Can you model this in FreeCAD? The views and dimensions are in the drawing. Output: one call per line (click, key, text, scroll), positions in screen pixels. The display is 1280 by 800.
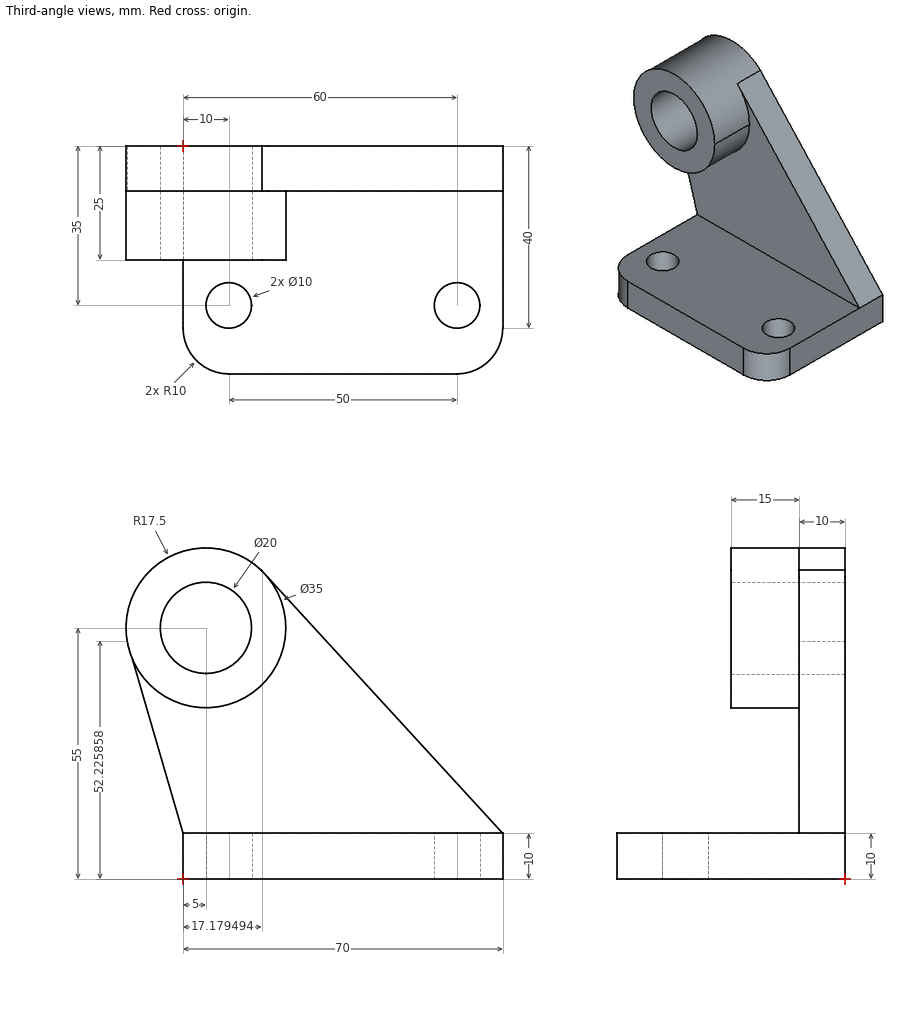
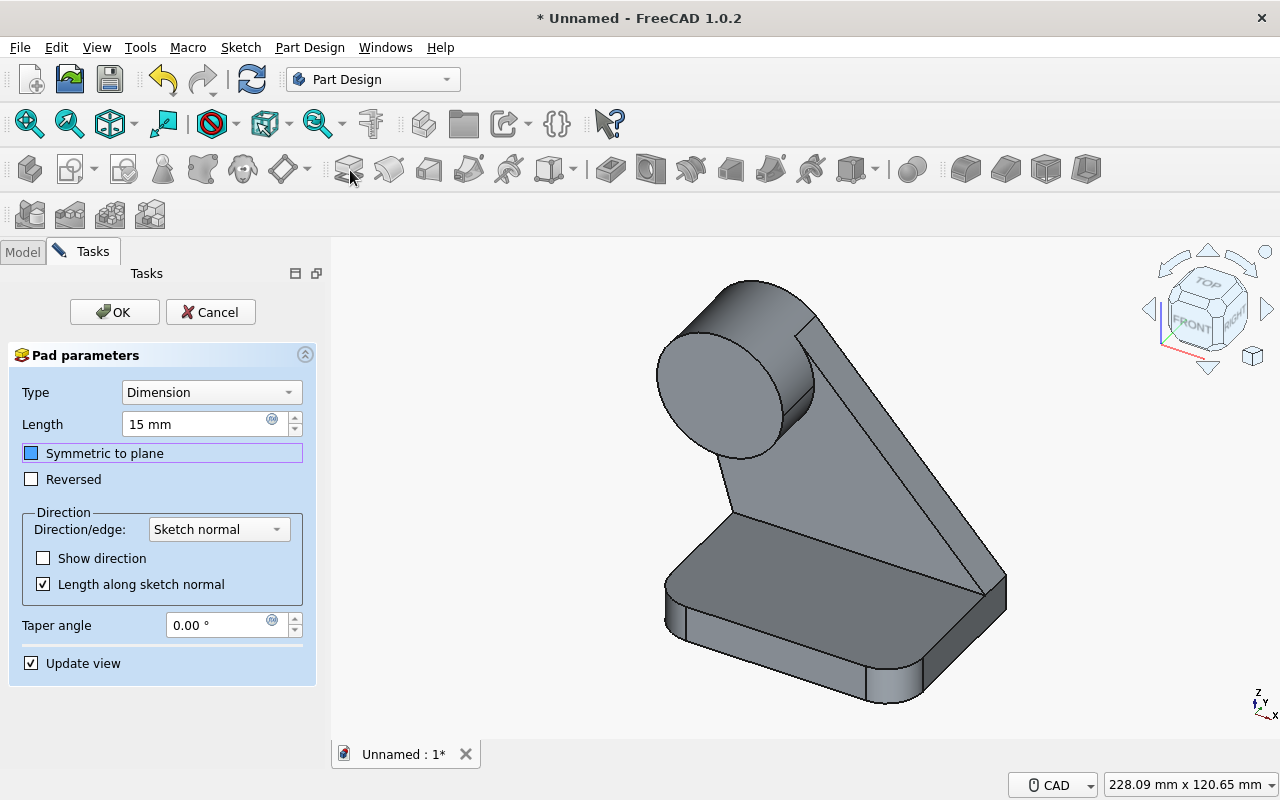
click(115, 312)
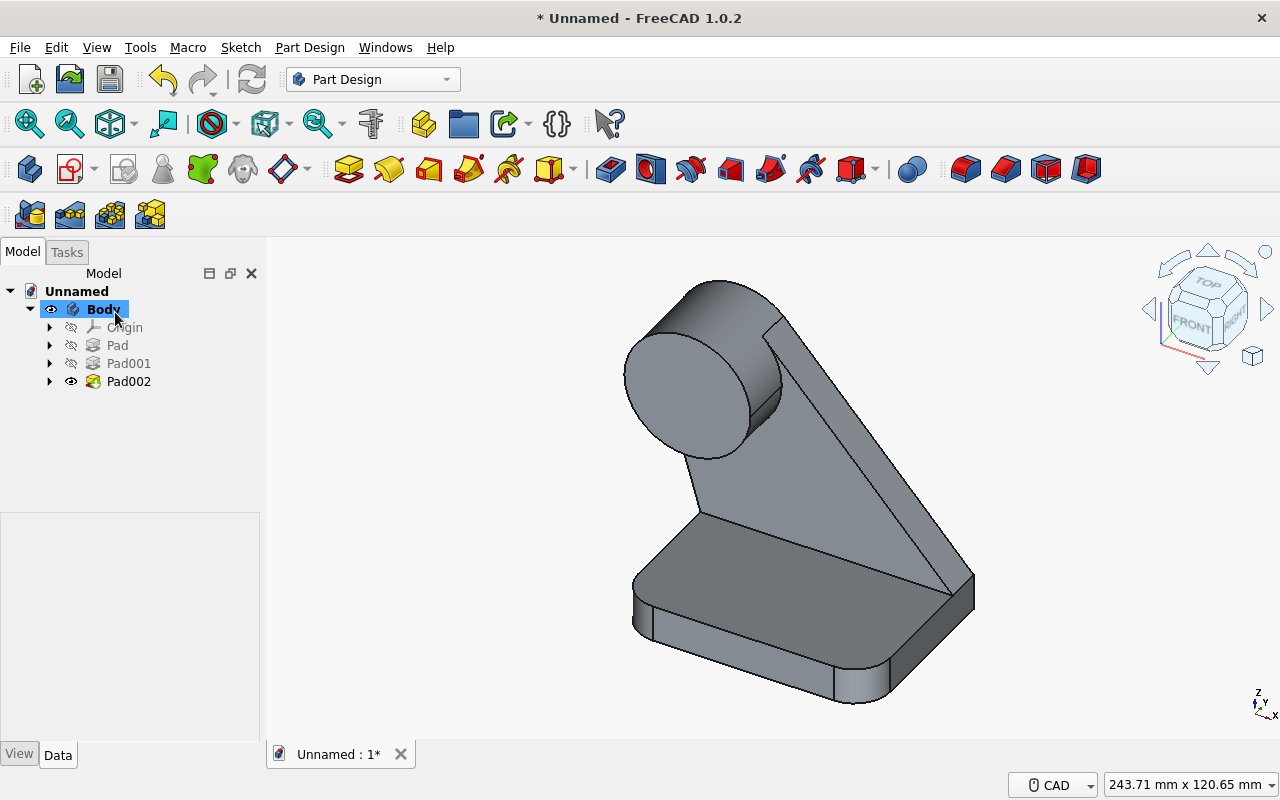
click(687, 395)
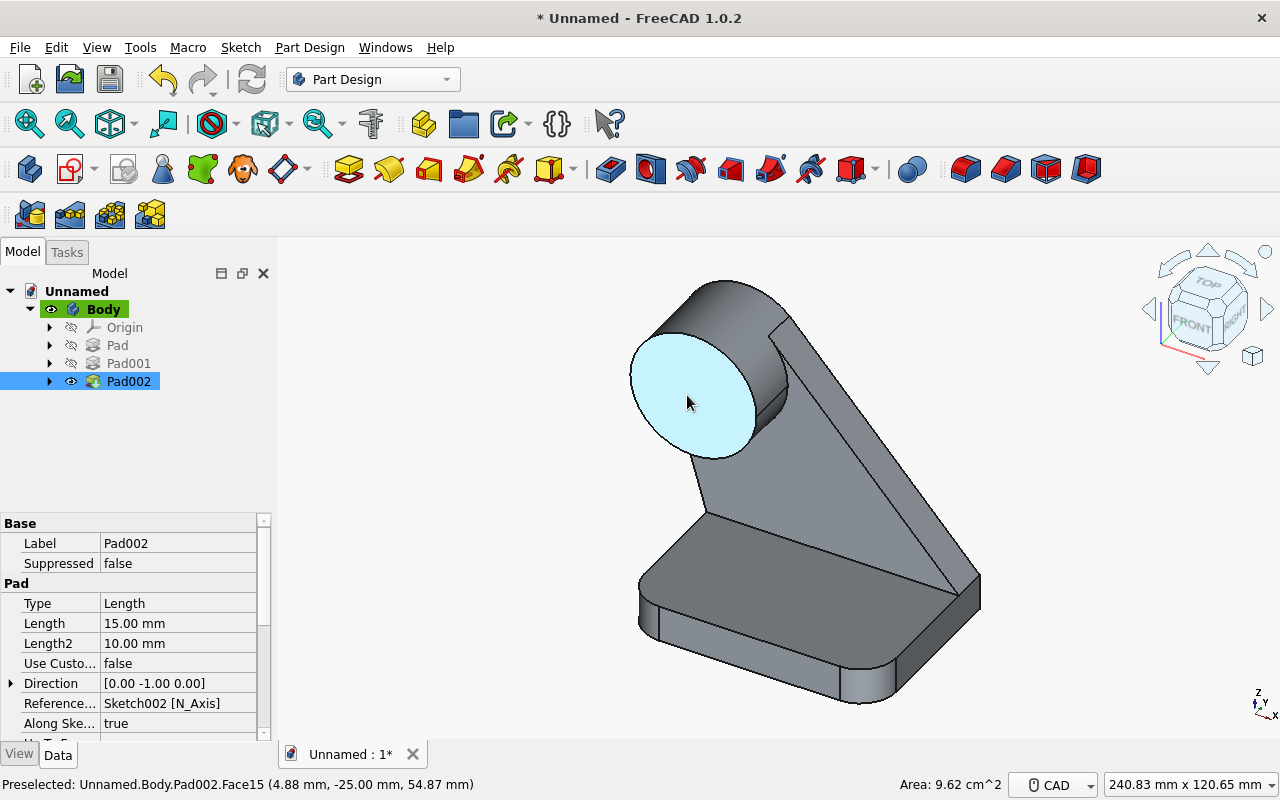
click(70, 170)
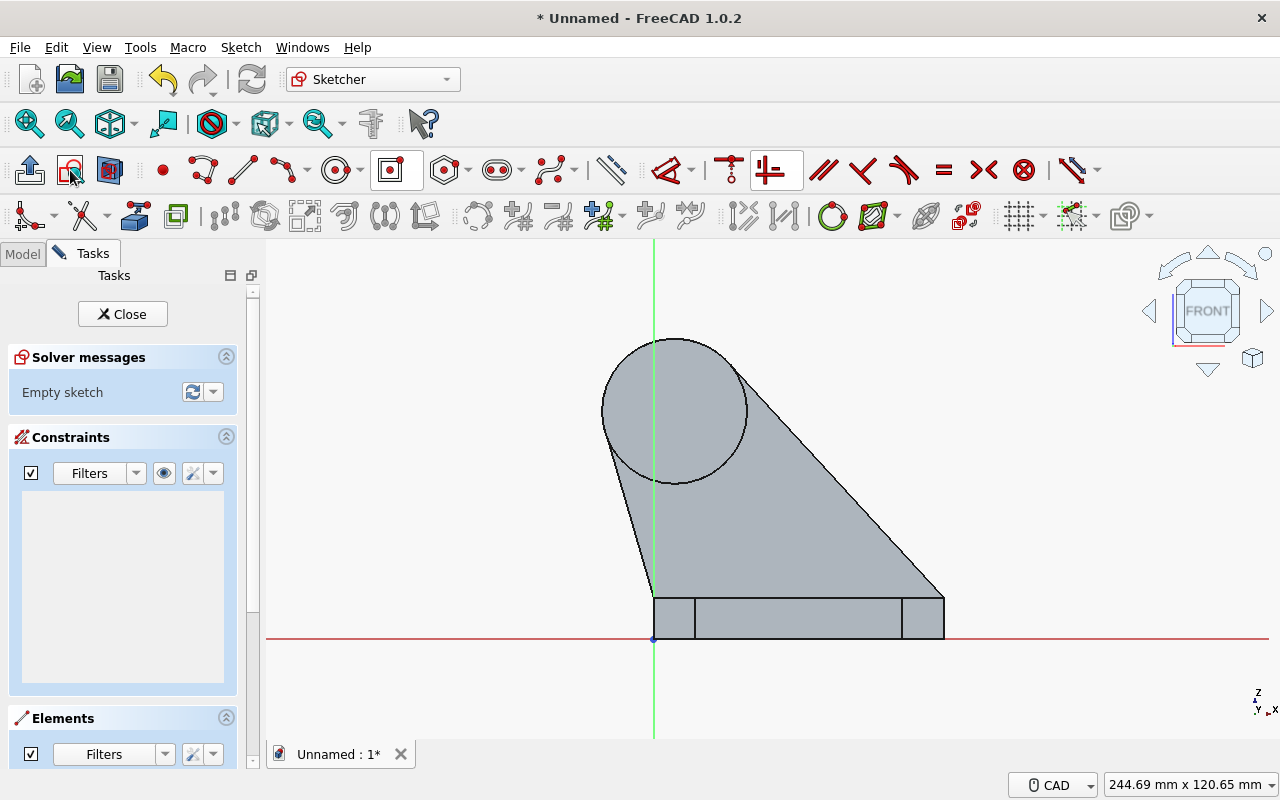
click(110, 170)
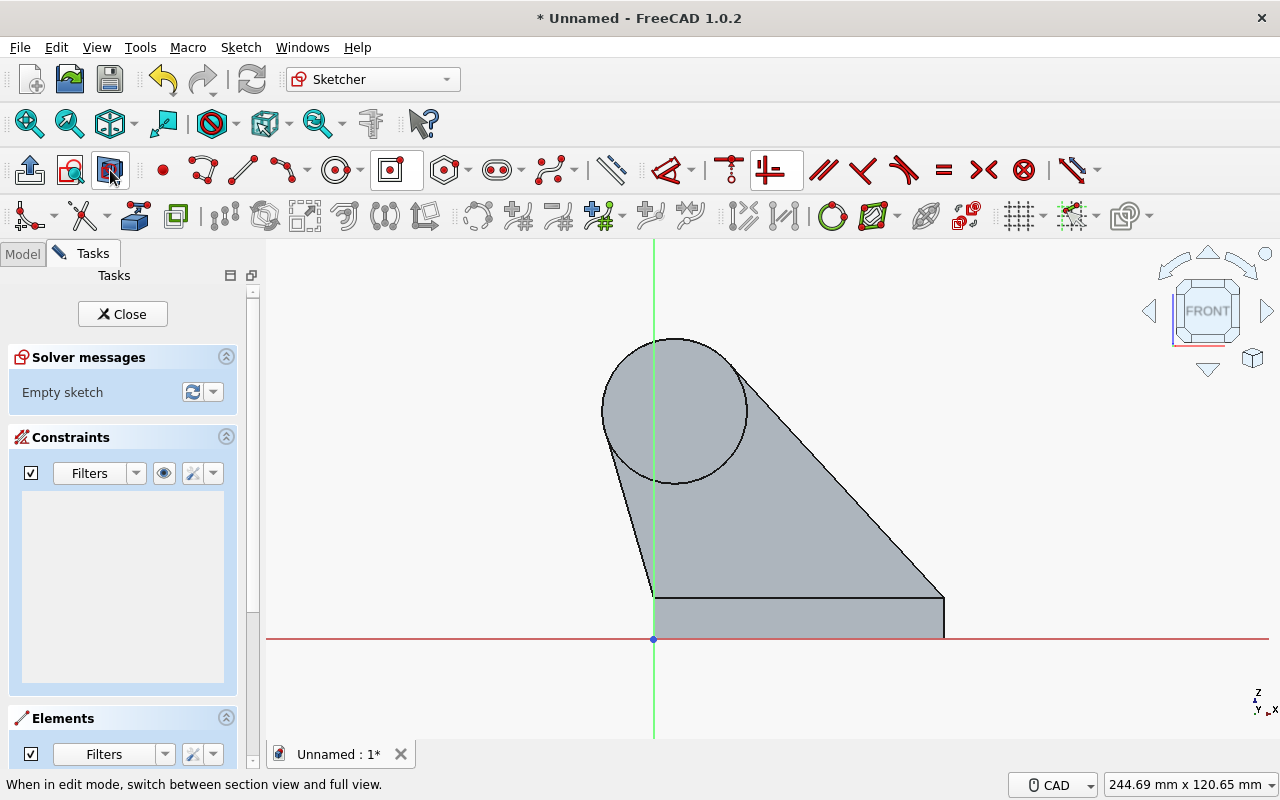
scroll(665, 386, up, 7)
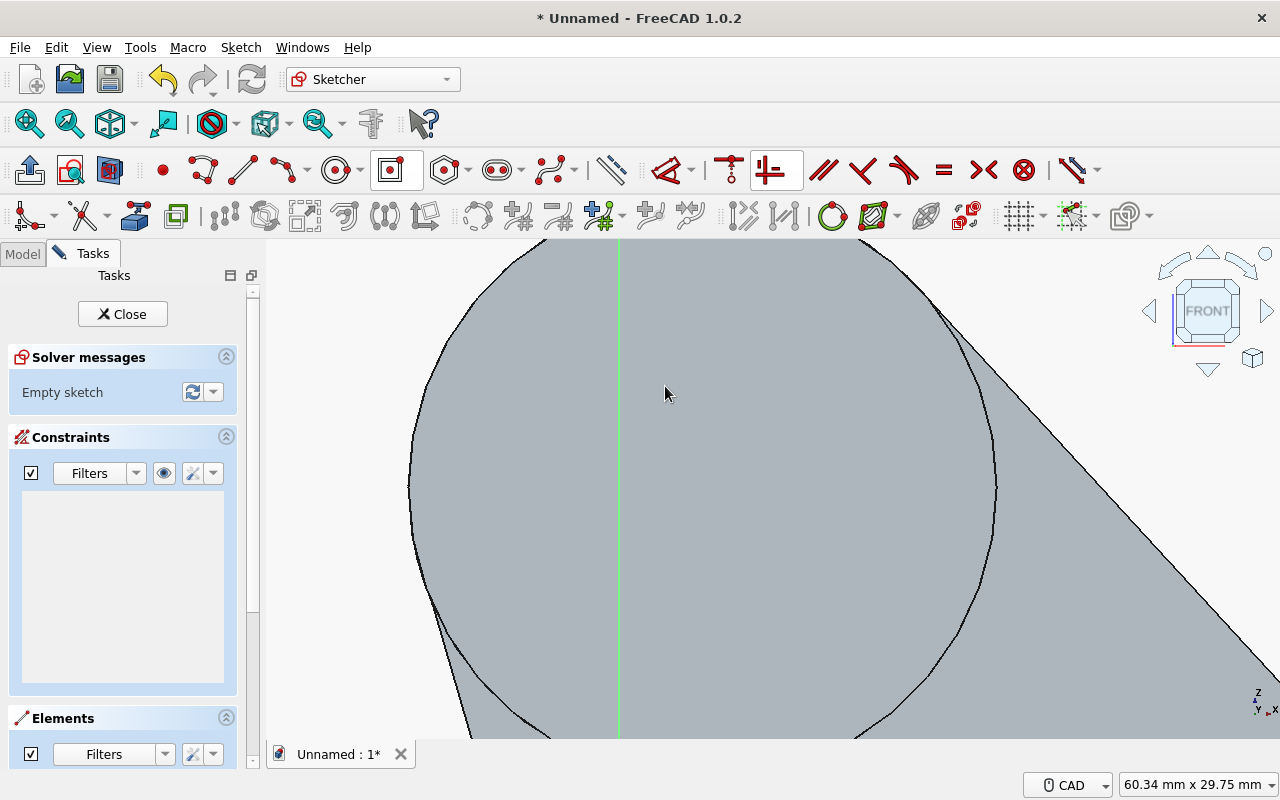
click(336, 170)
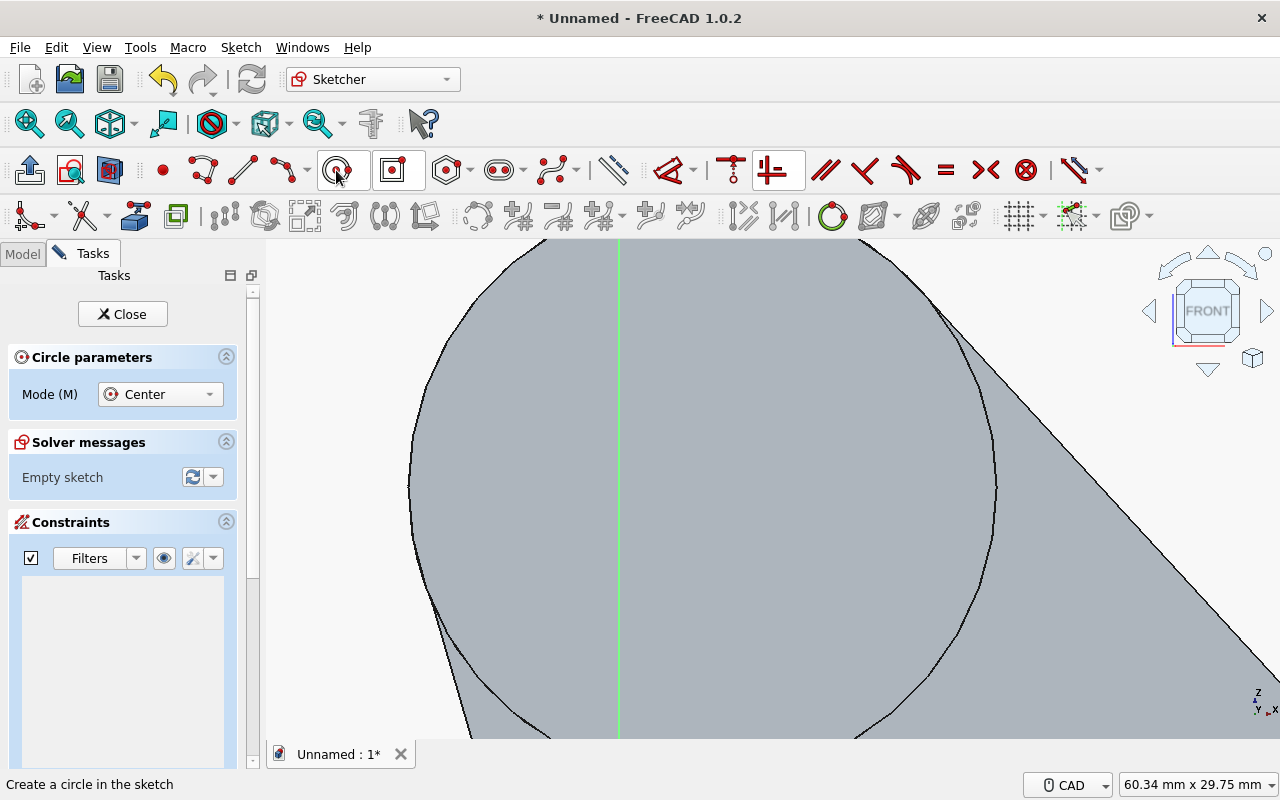
click(703, 487)
click(821, 369)
key(Escape)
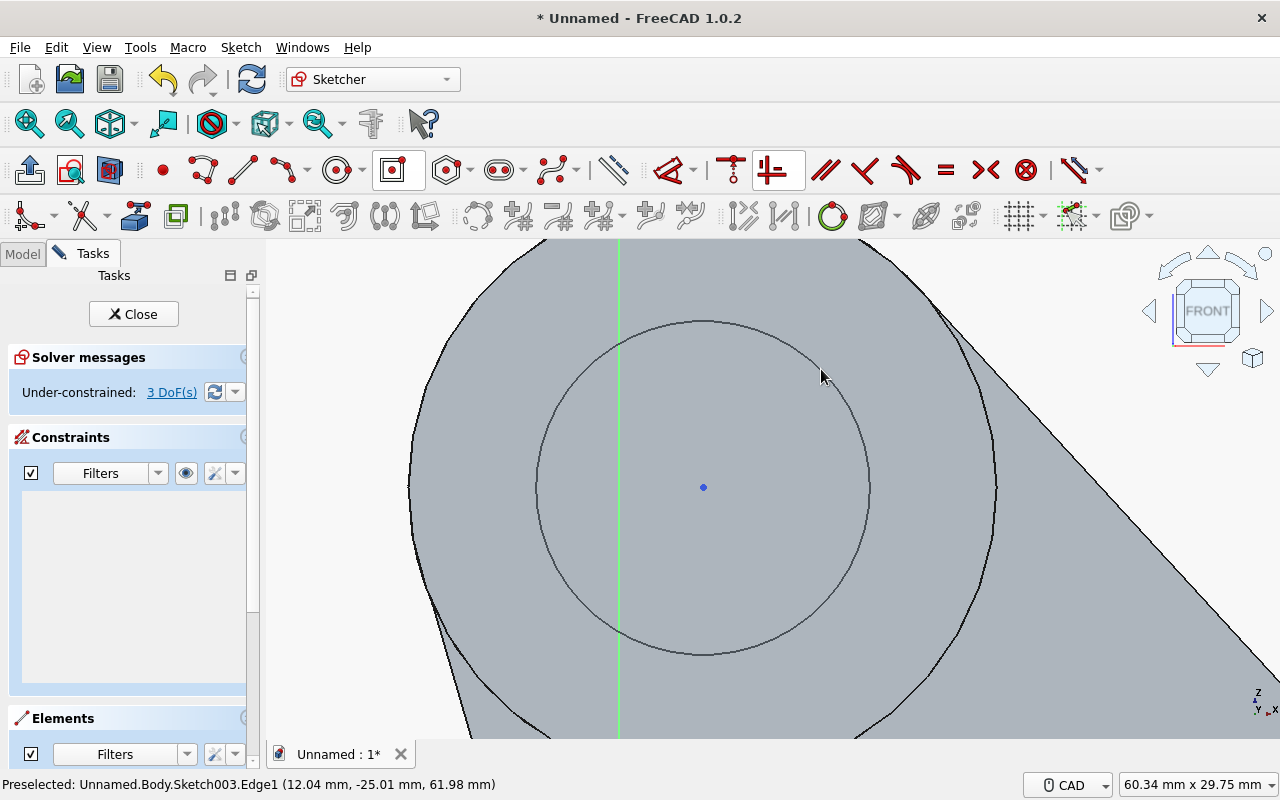
click(668, 170)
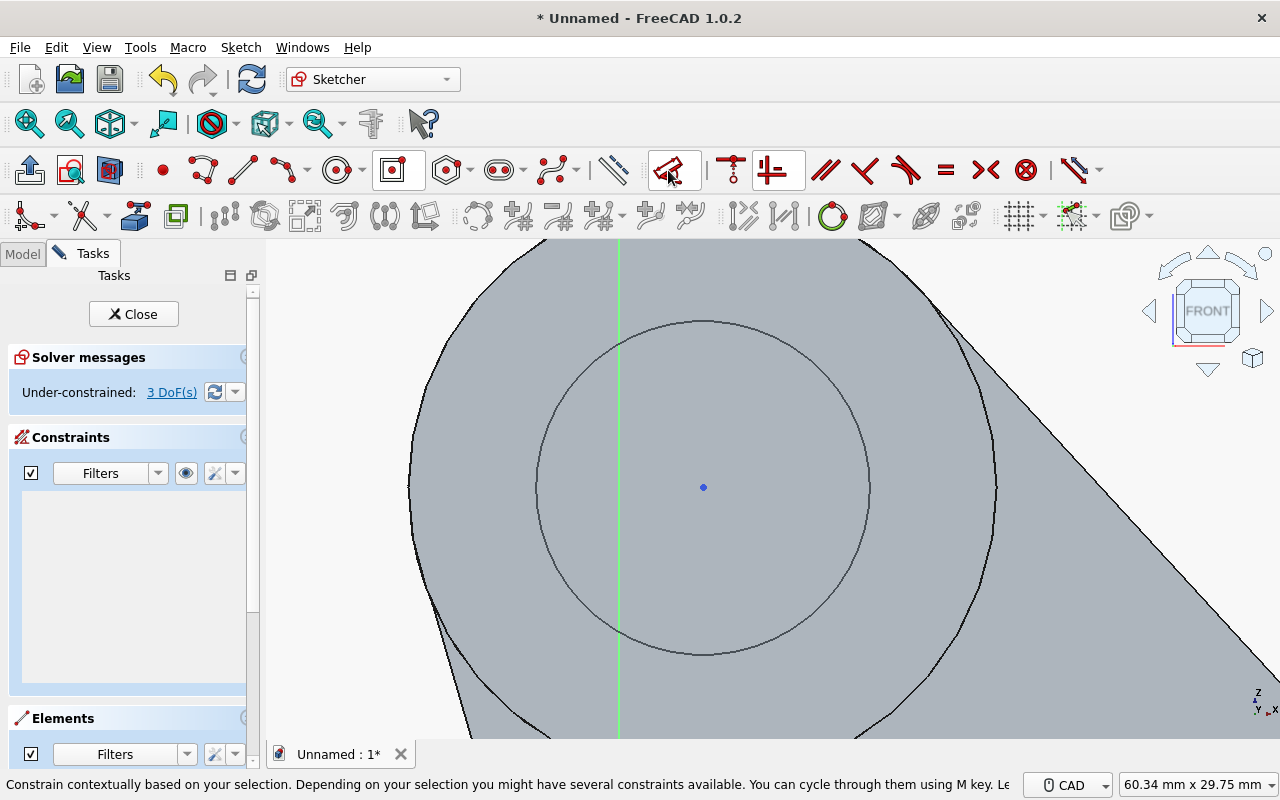
click(821, 370)
click(844, 347)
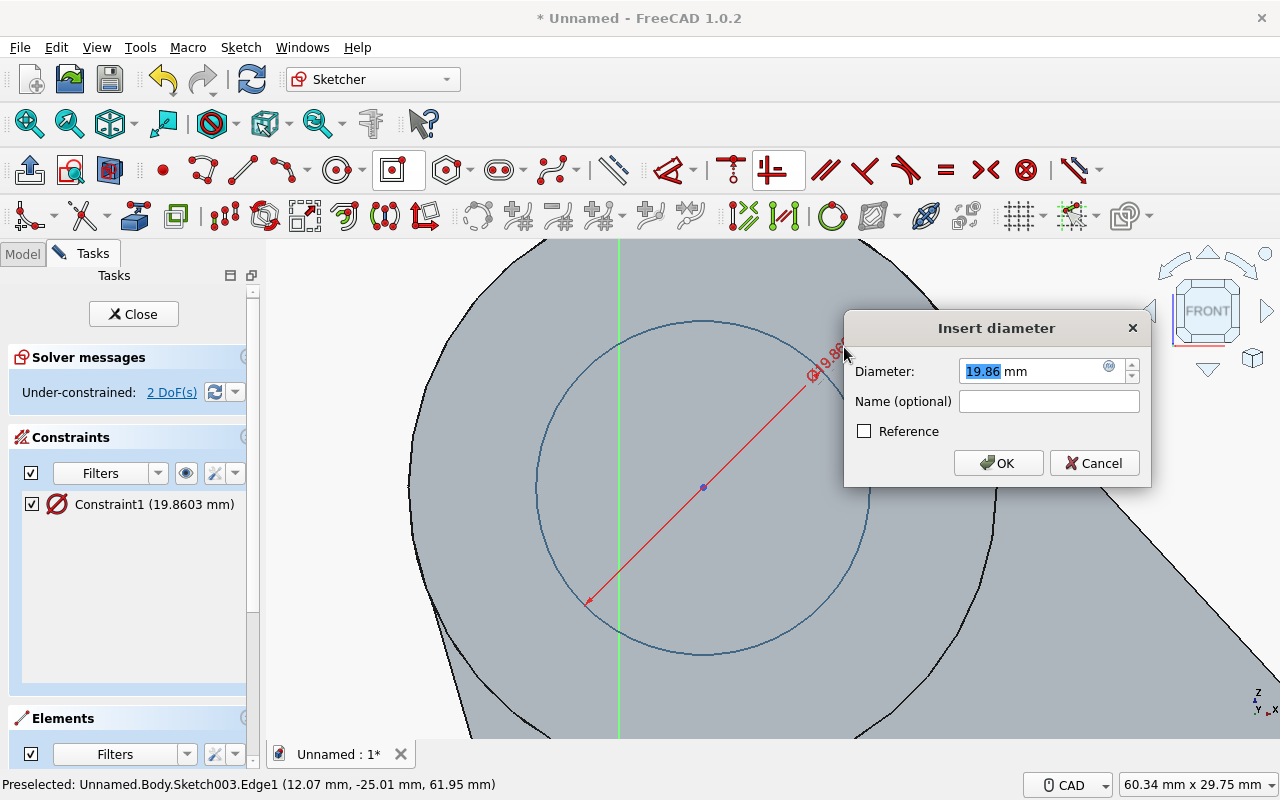
text(20)
key(Return)